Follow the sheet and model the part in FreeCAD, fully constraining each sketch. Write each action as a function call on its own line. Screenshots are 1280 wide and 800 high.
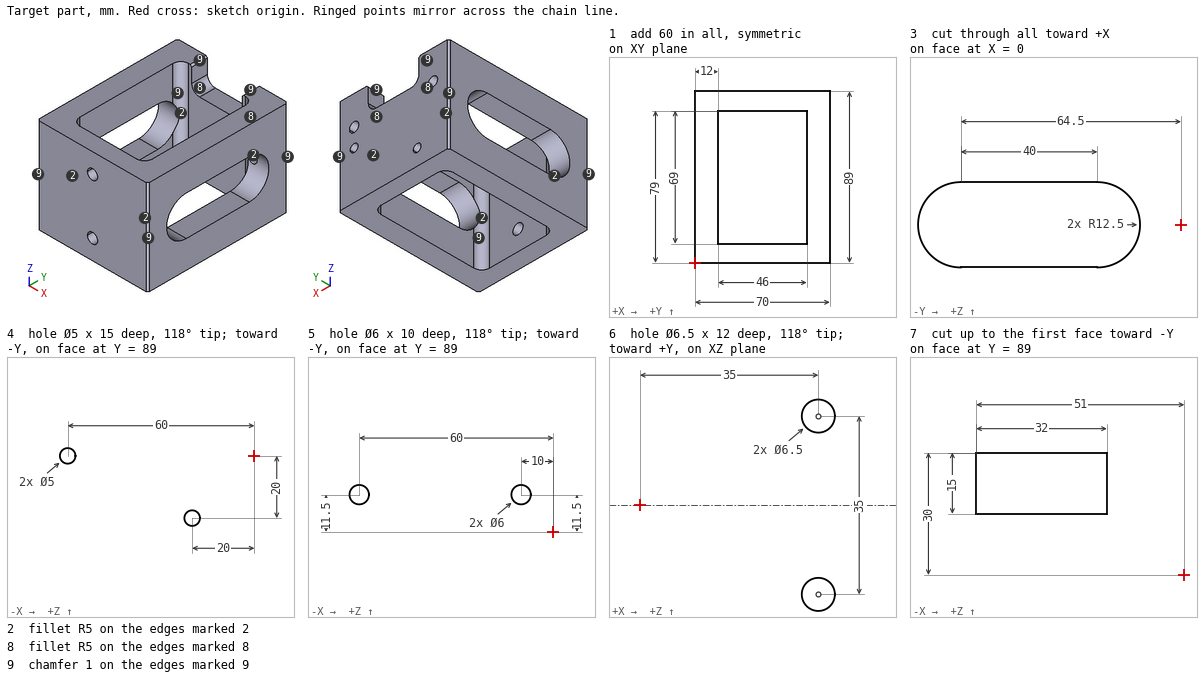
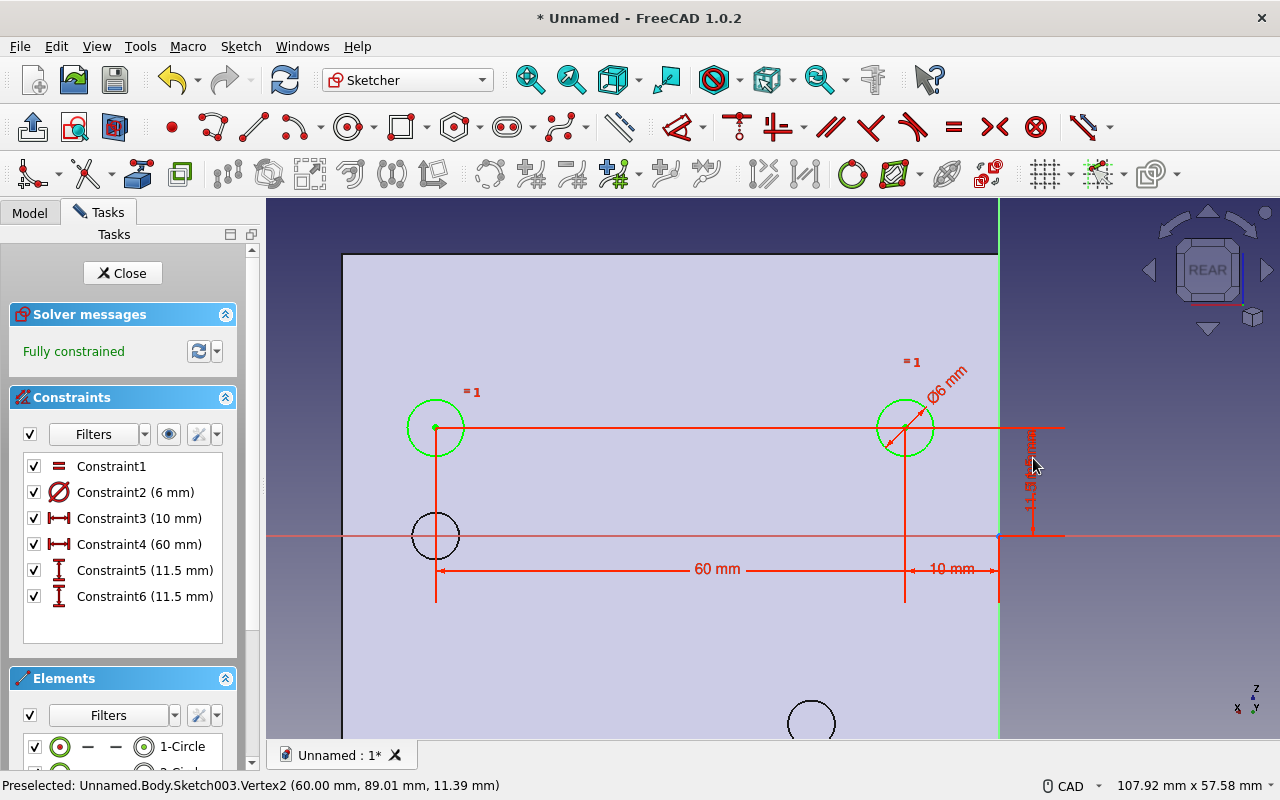
click(123, 273)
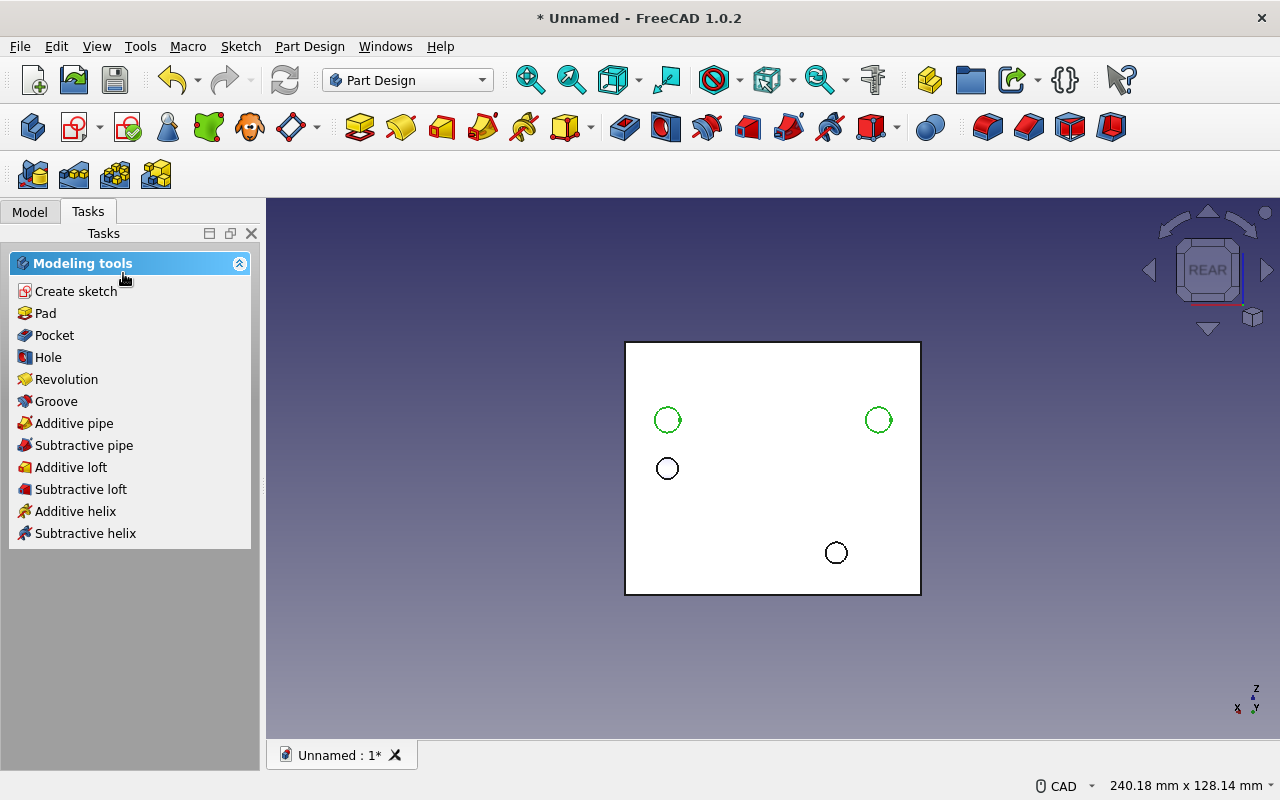
click(666, 128)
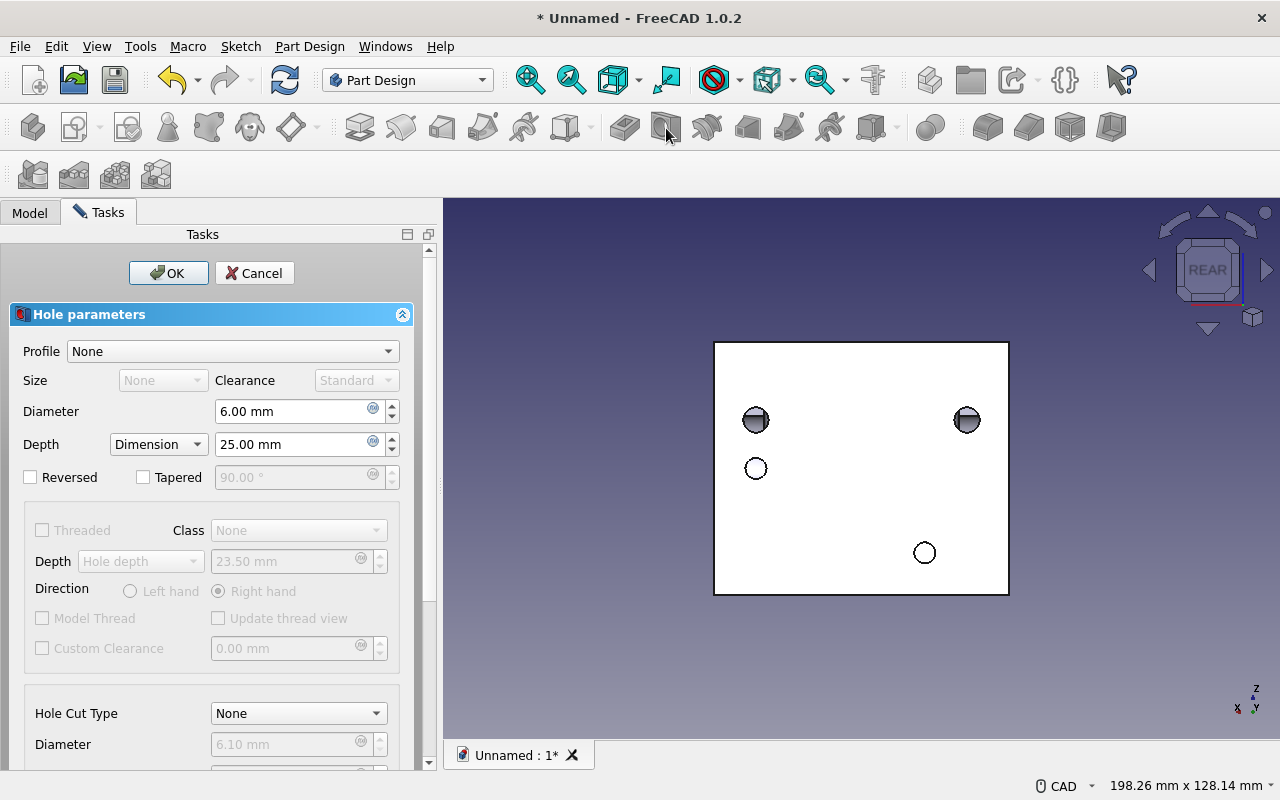
triple_click(300, 412)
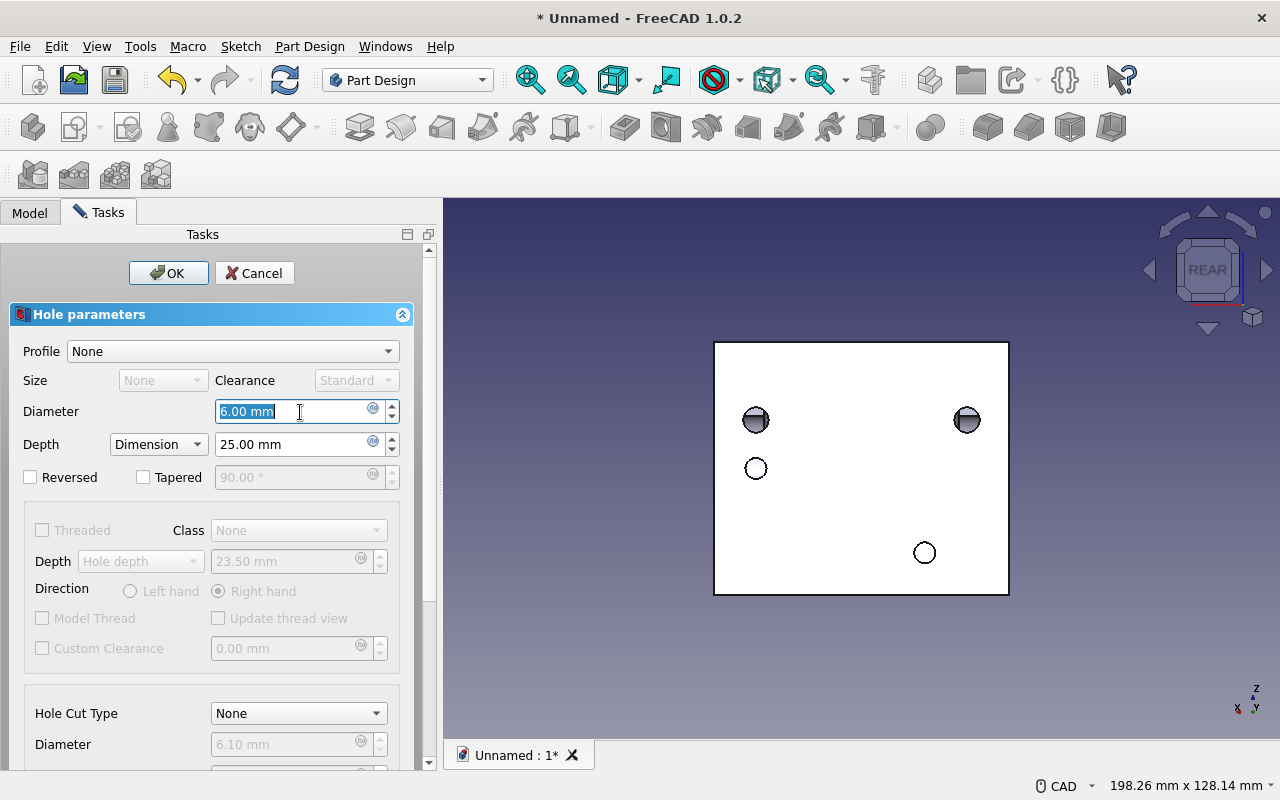
text(6)
key(Tab)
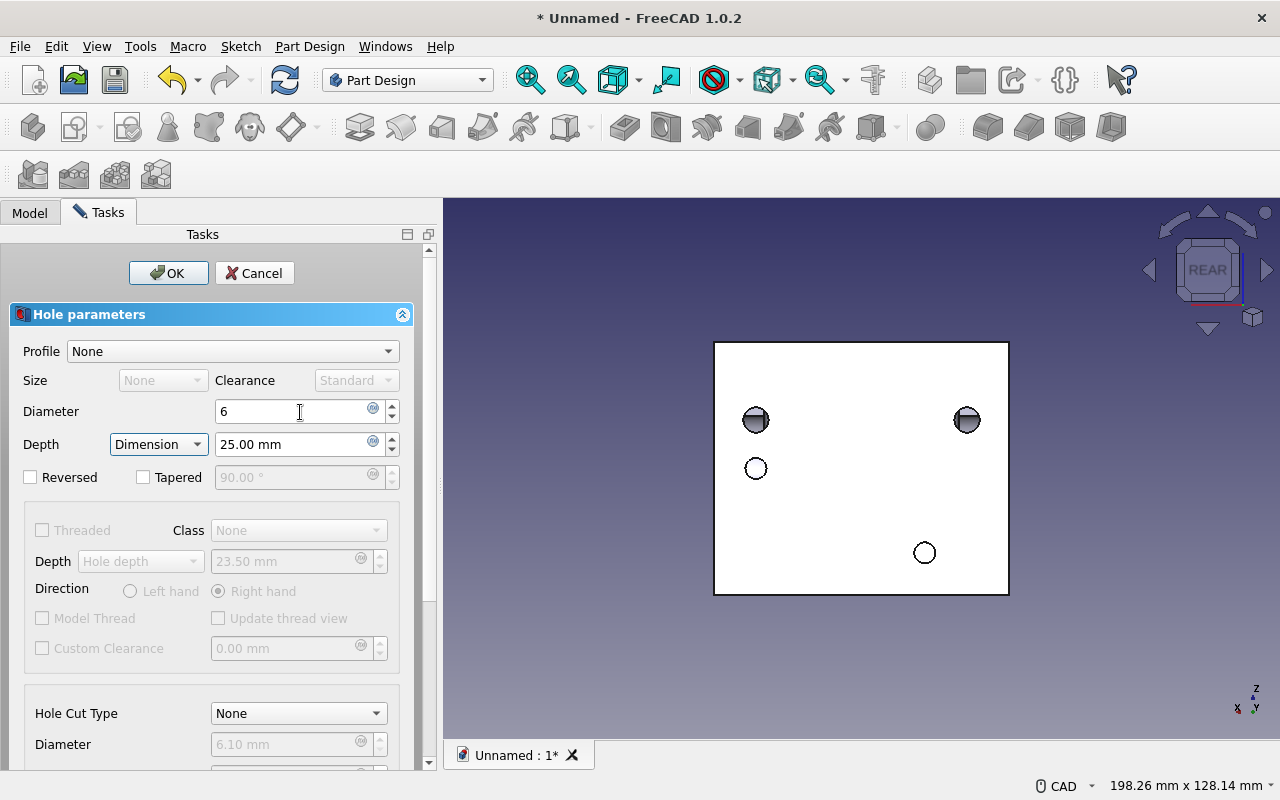
triple_click(300, 444)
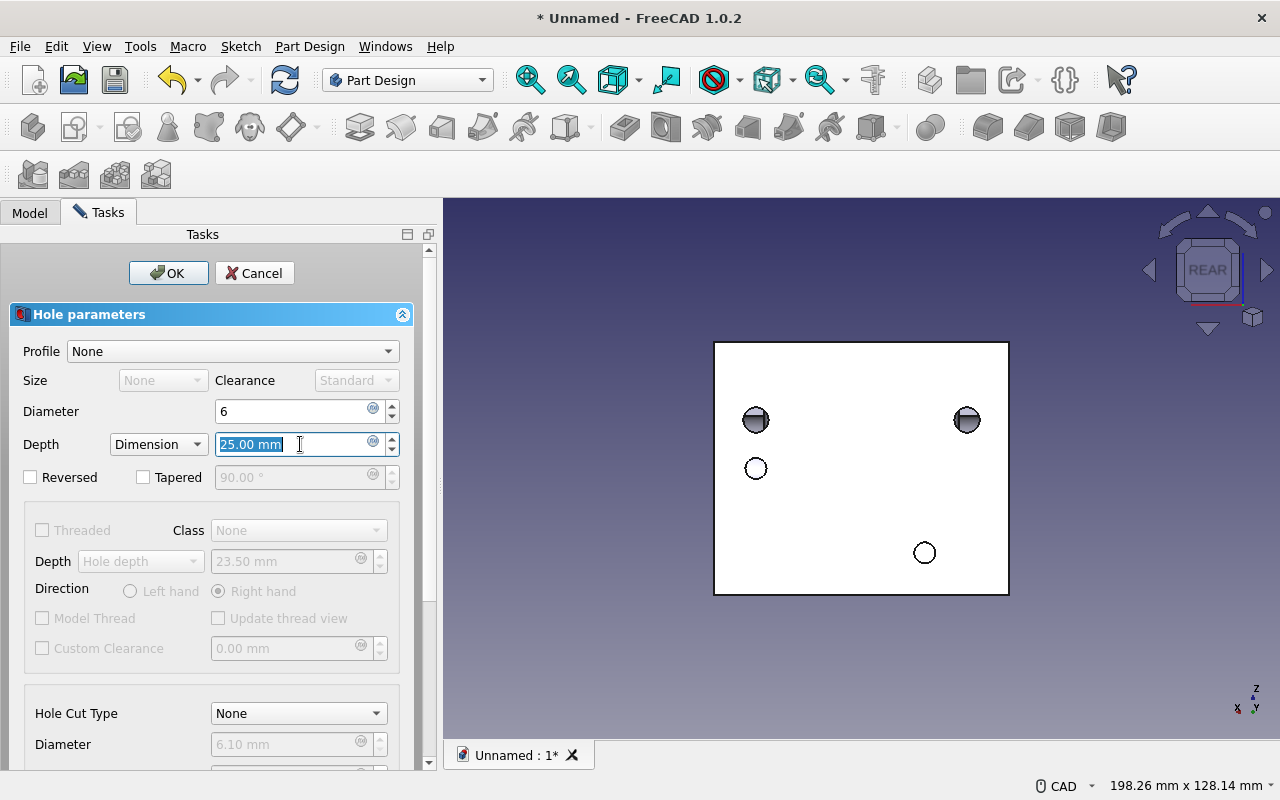
text(10)
key(Tab)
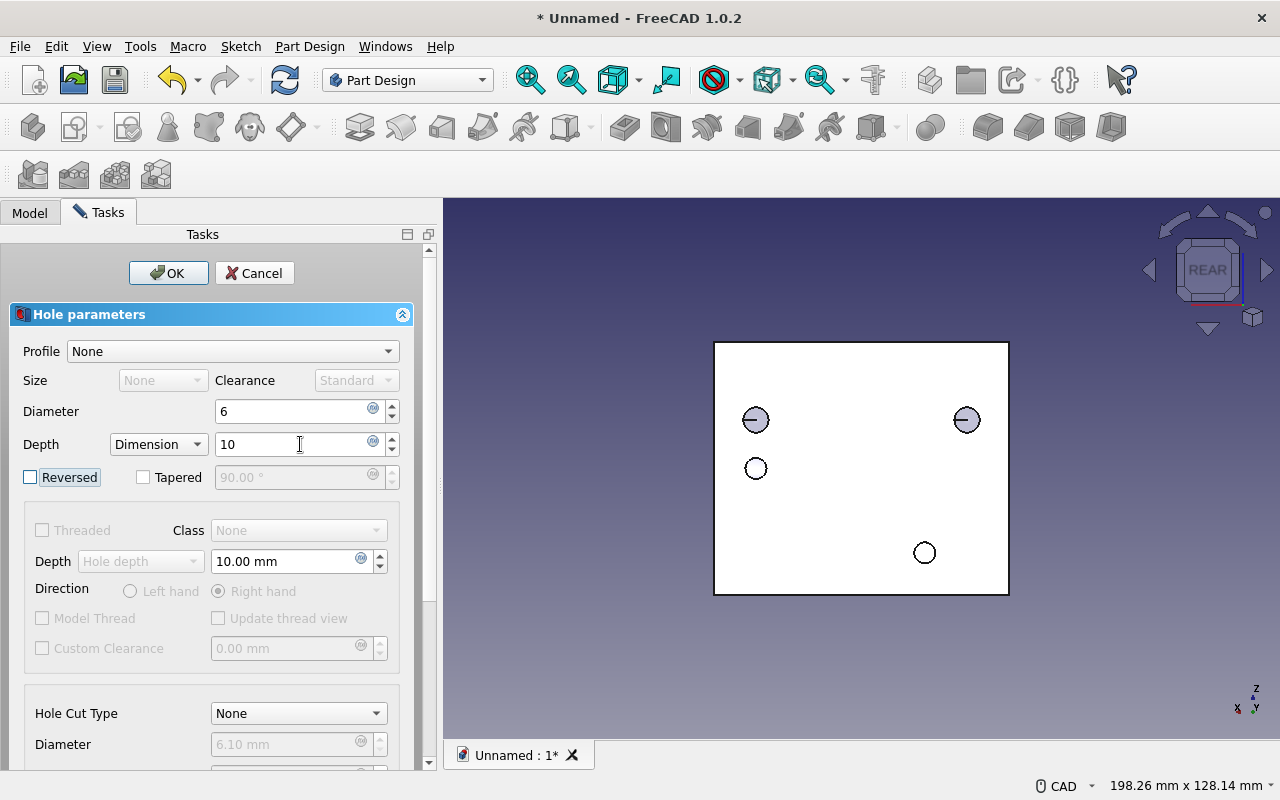
click(169, 273)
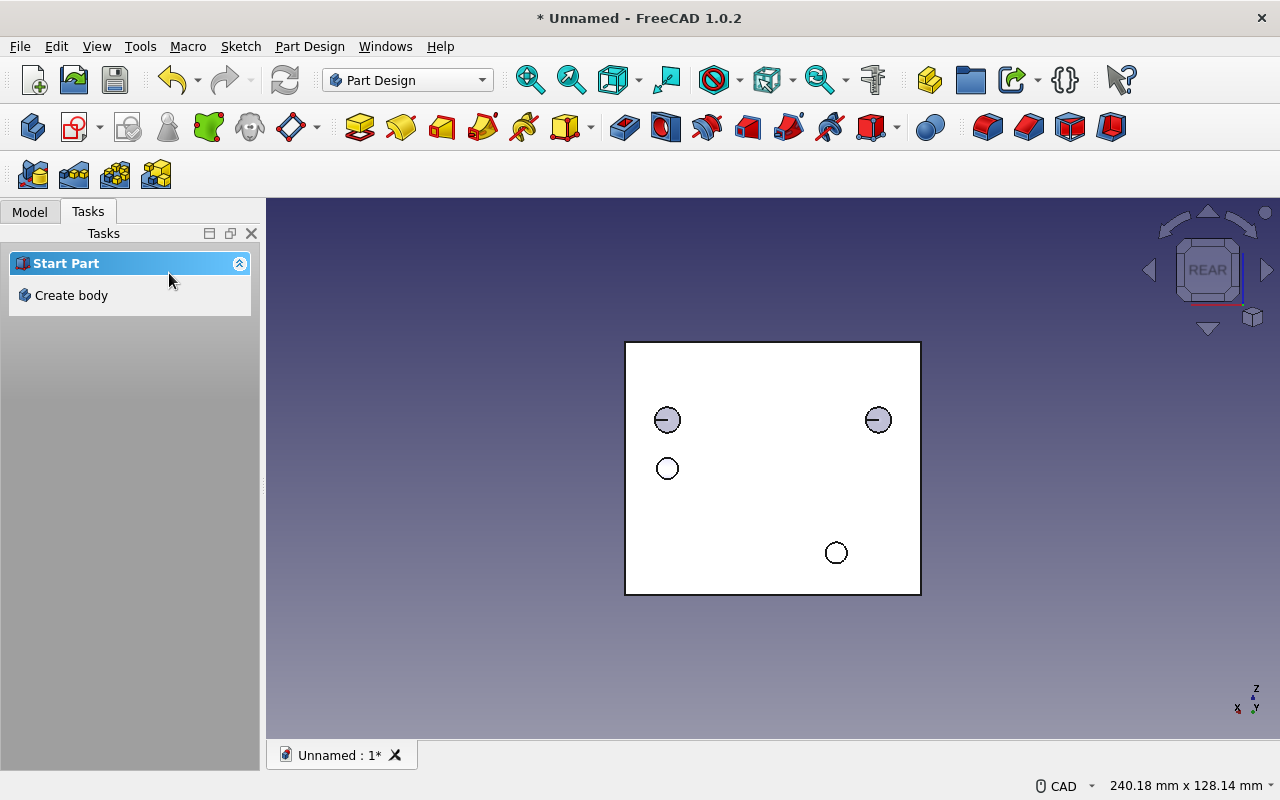
click(74, 128)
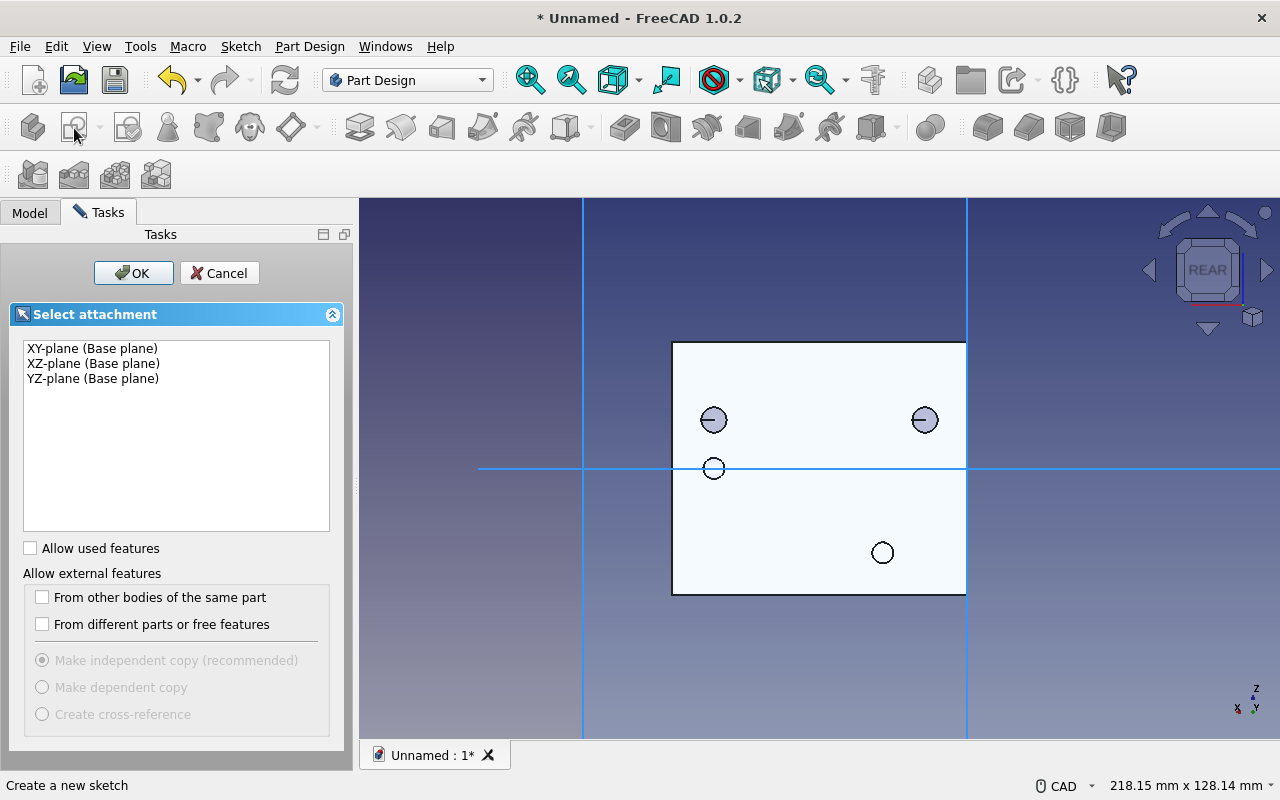
click(84, 364)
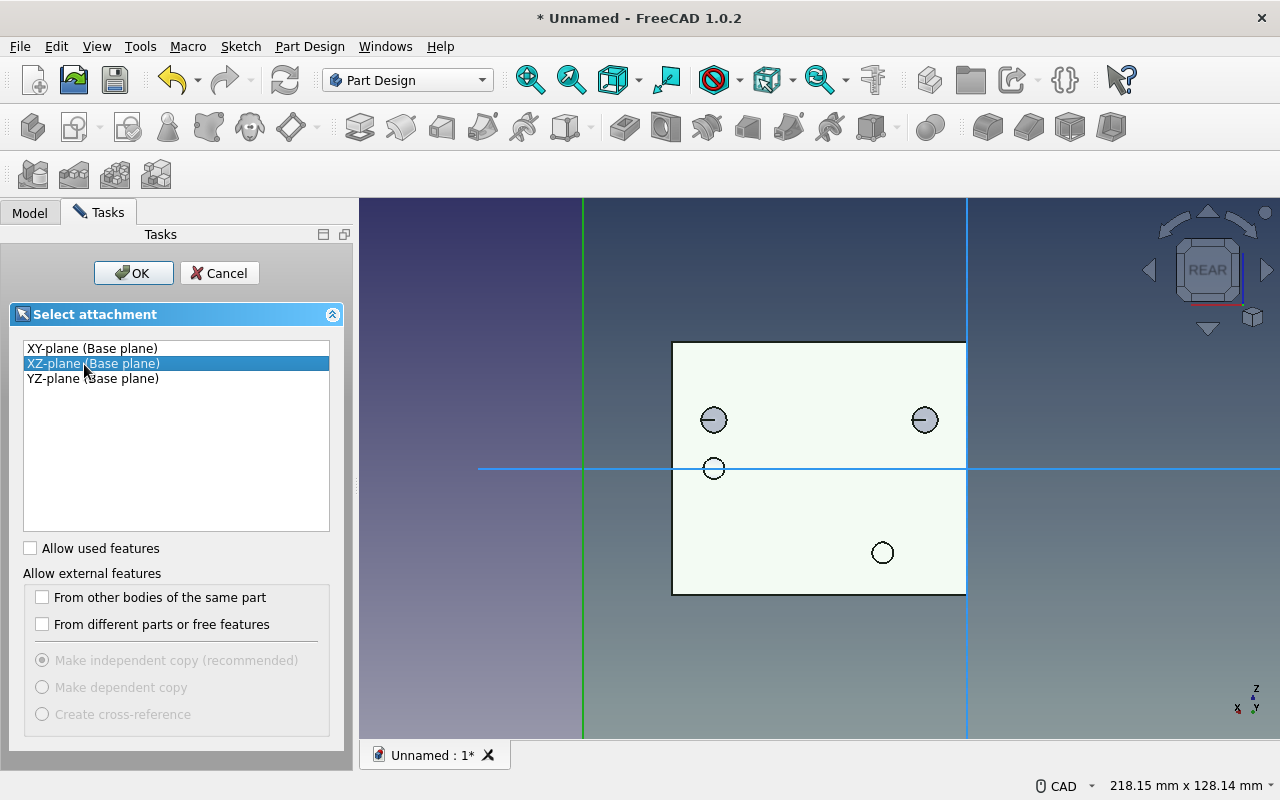
click(134, 273)